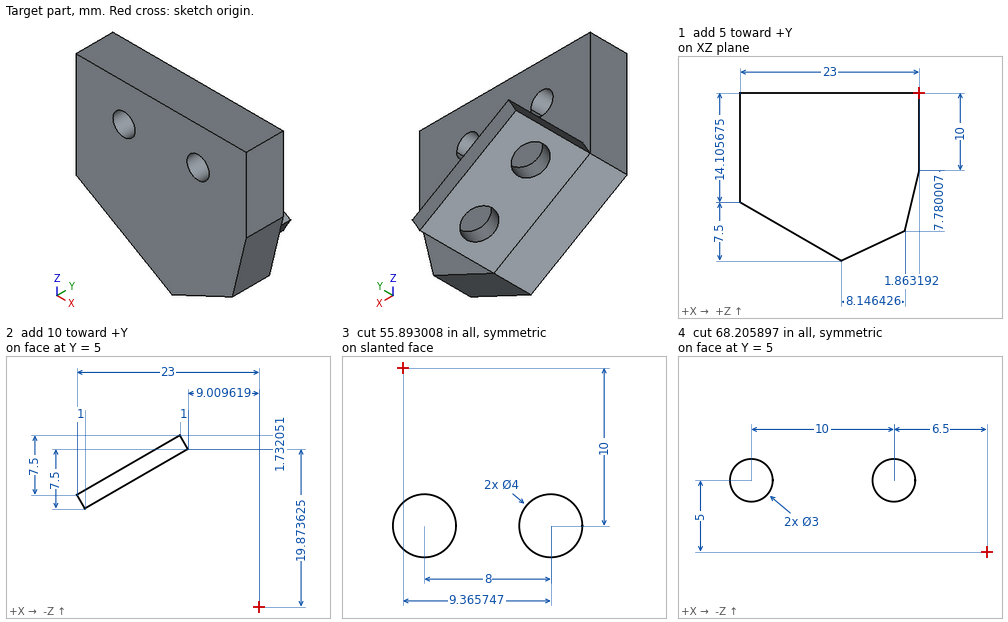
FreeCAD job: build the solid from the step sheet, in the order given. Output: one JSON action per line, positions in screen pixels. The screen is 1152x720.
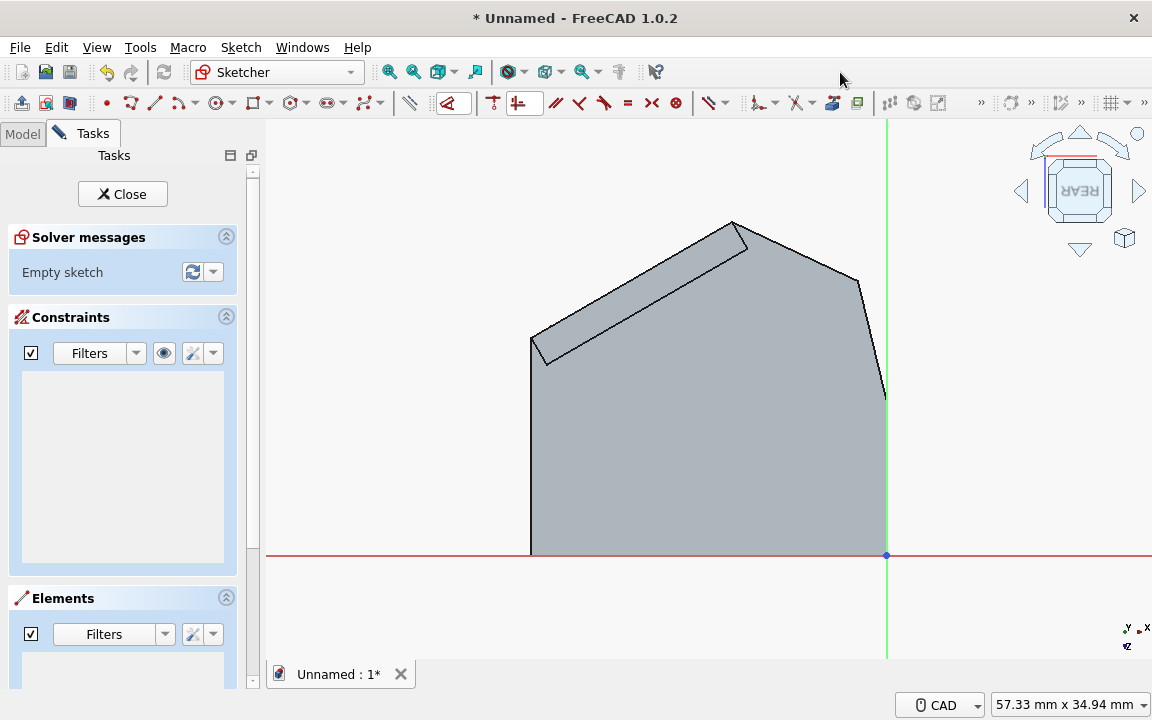
{"action": "scroll", "coordinate": [878, 631], "scroll_direction": "up", "scroll_amount": 3}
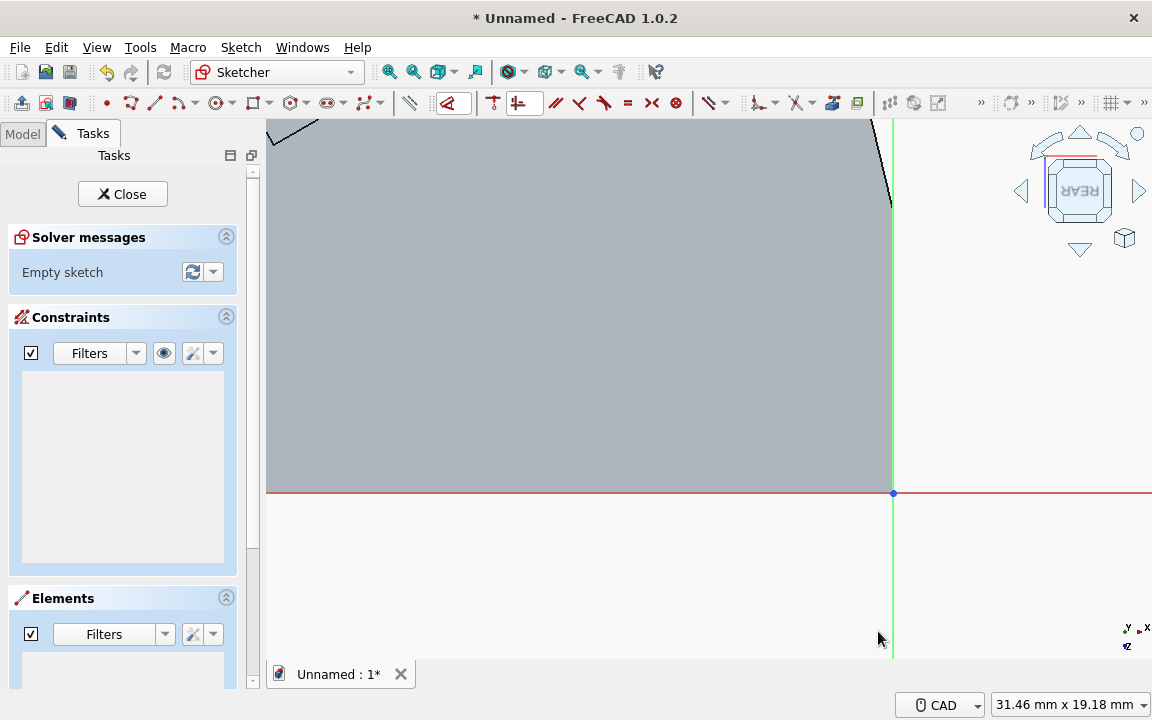
{"action": "left_click", "coordinate": [216, 104]}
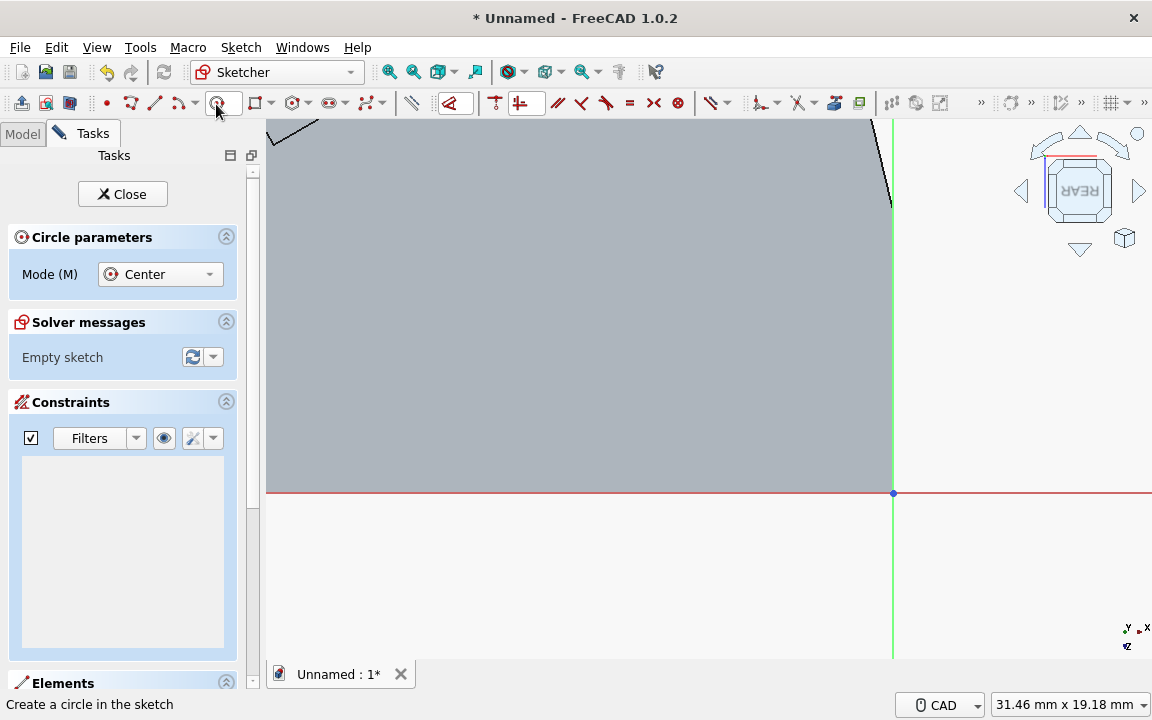
{"action": "left_click", "coordinate": [429, 353]}
{"action": "mouse_move", "coordinate": [459, 323]}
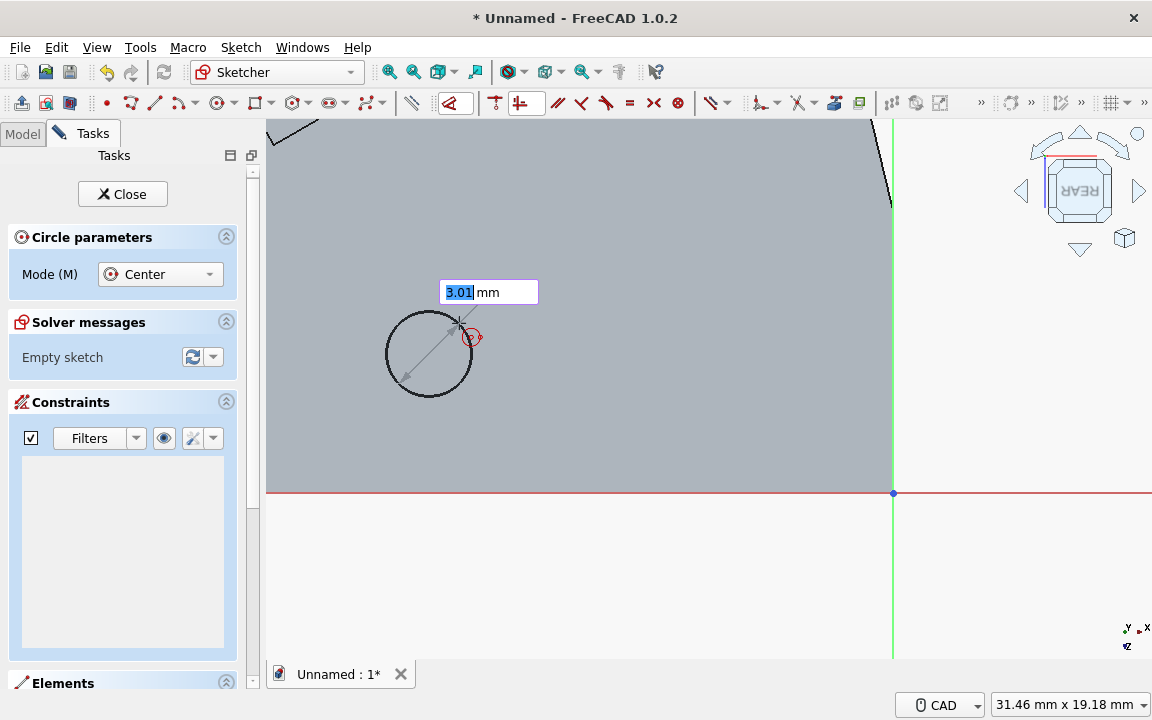
{"action": "type", "text": "3"}
{"action": "key", "text": "Return"}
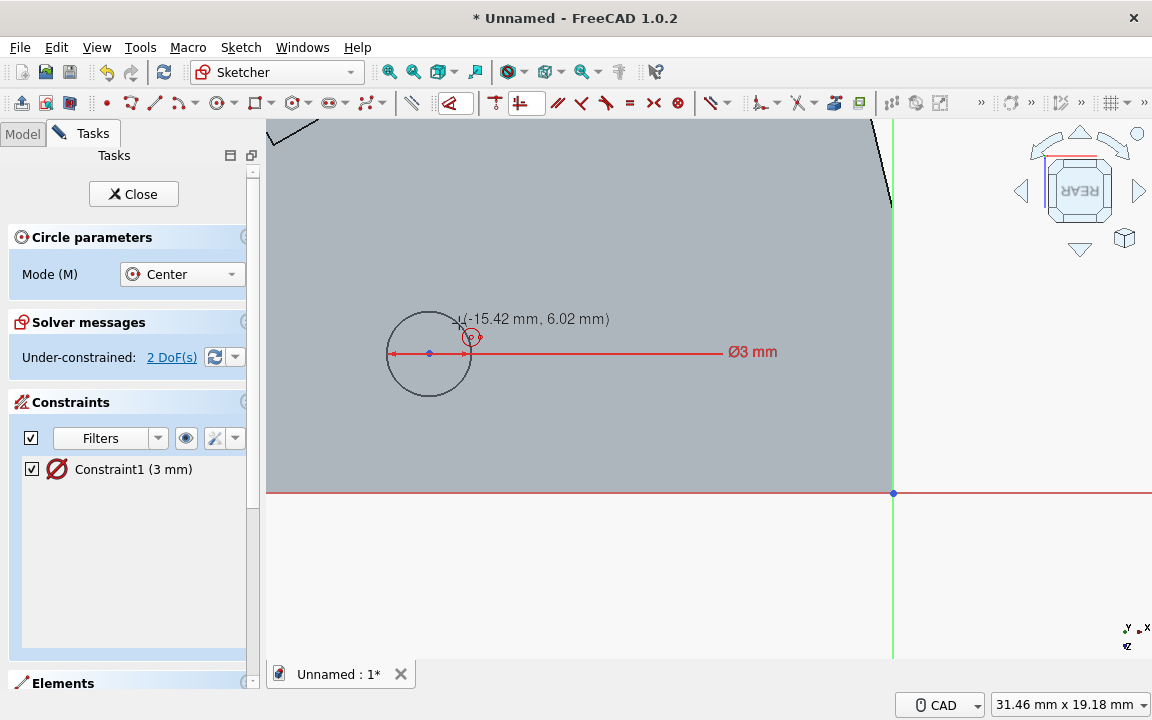
{"action": "left_click", "coordinate": [710, 353]}
{"action": "mouse_move", "coordinate": [740, 323]}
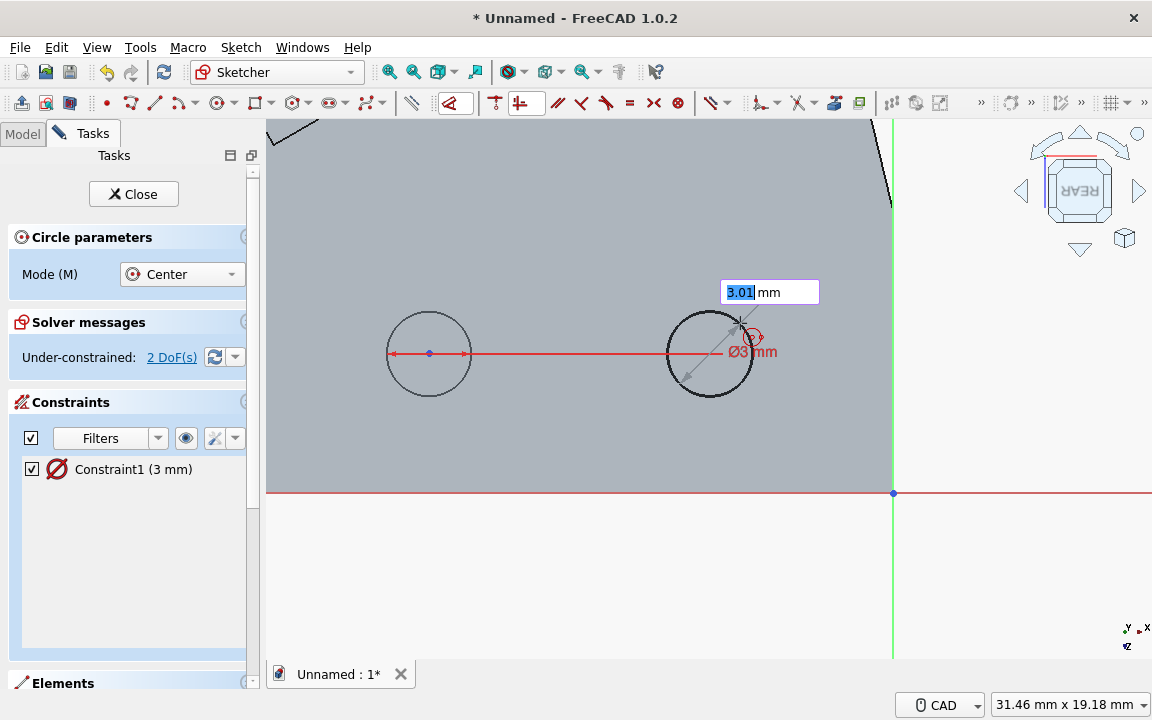
{"action": "type", "text": "3"}
{"action": "key", "text": "Return"}
{"action": "key", "text": "Escape"}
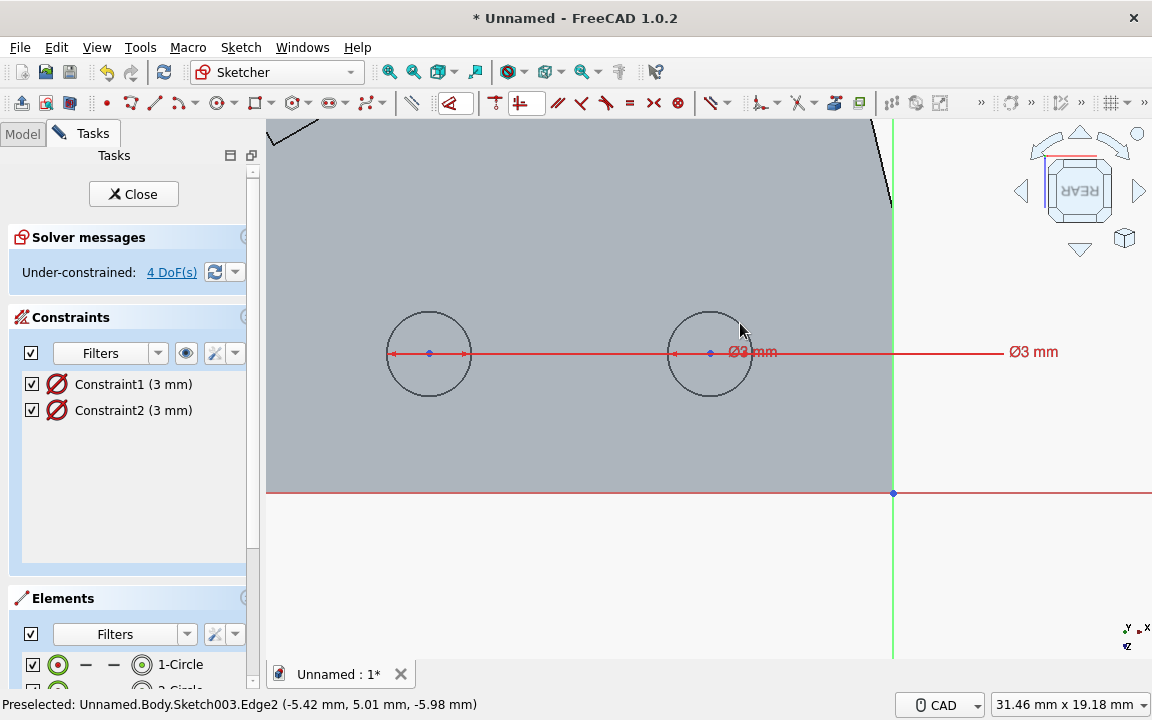
{"action": "left_click", "coordinate": [429, 354]}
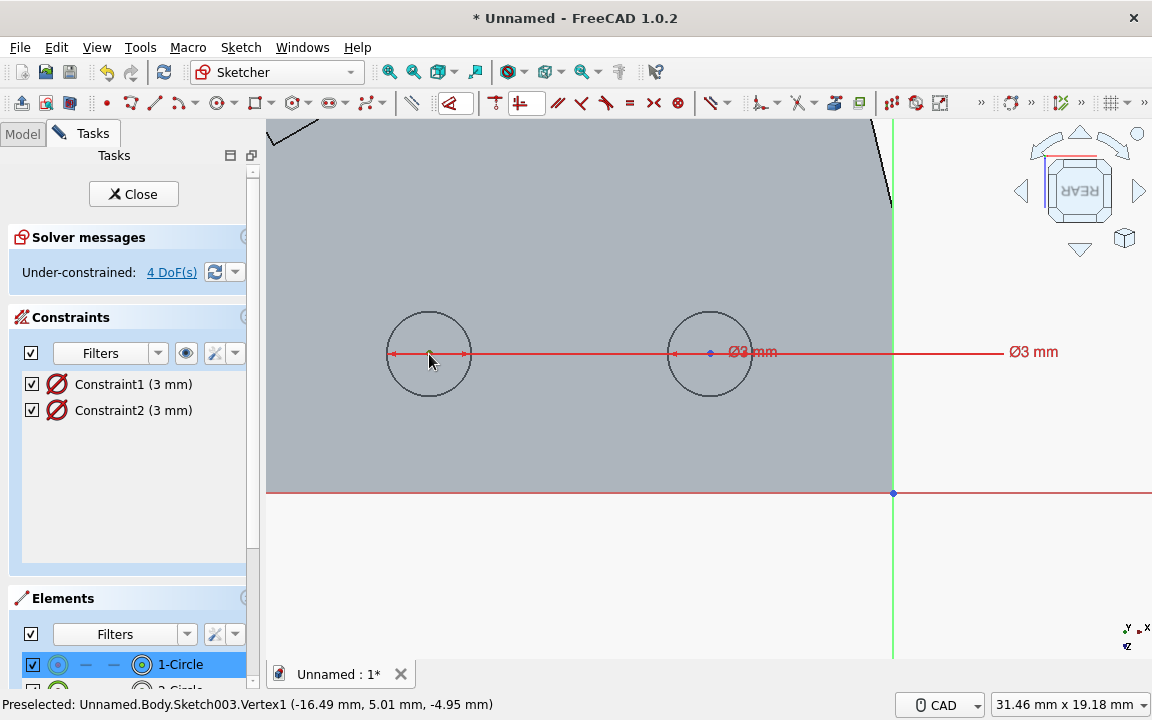
{"action": "left_click", "coordinate": [710, 354]}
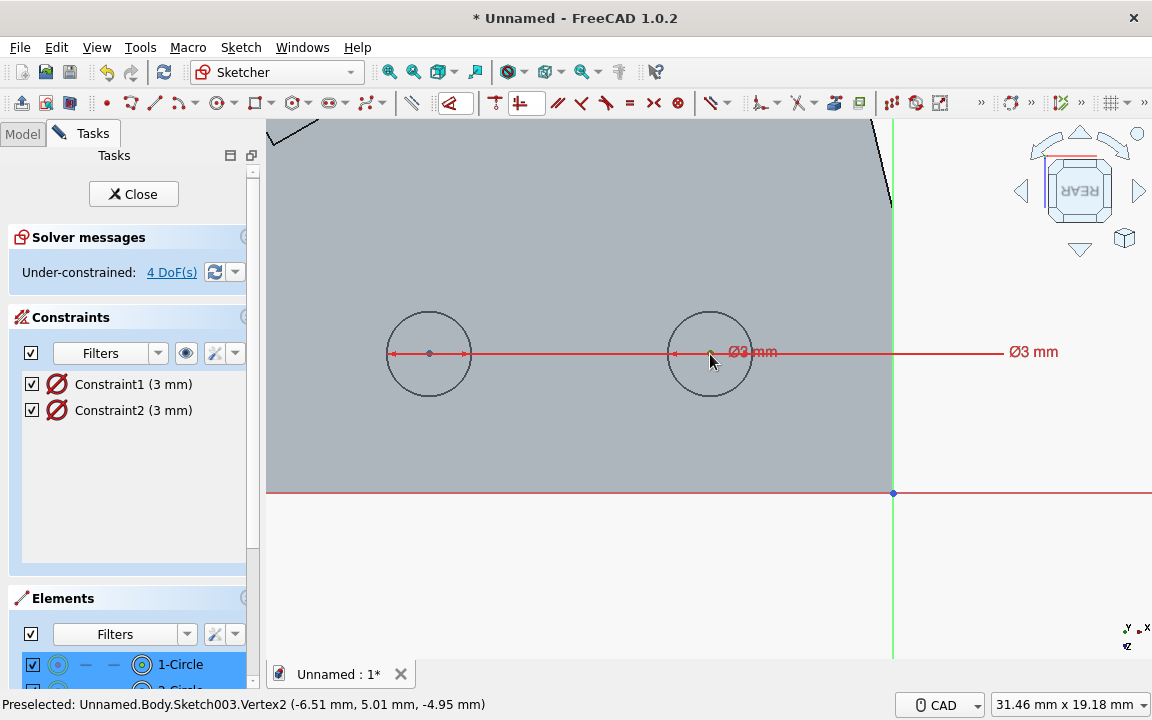
{"action": "left_click", "coordinate": [540, 104]}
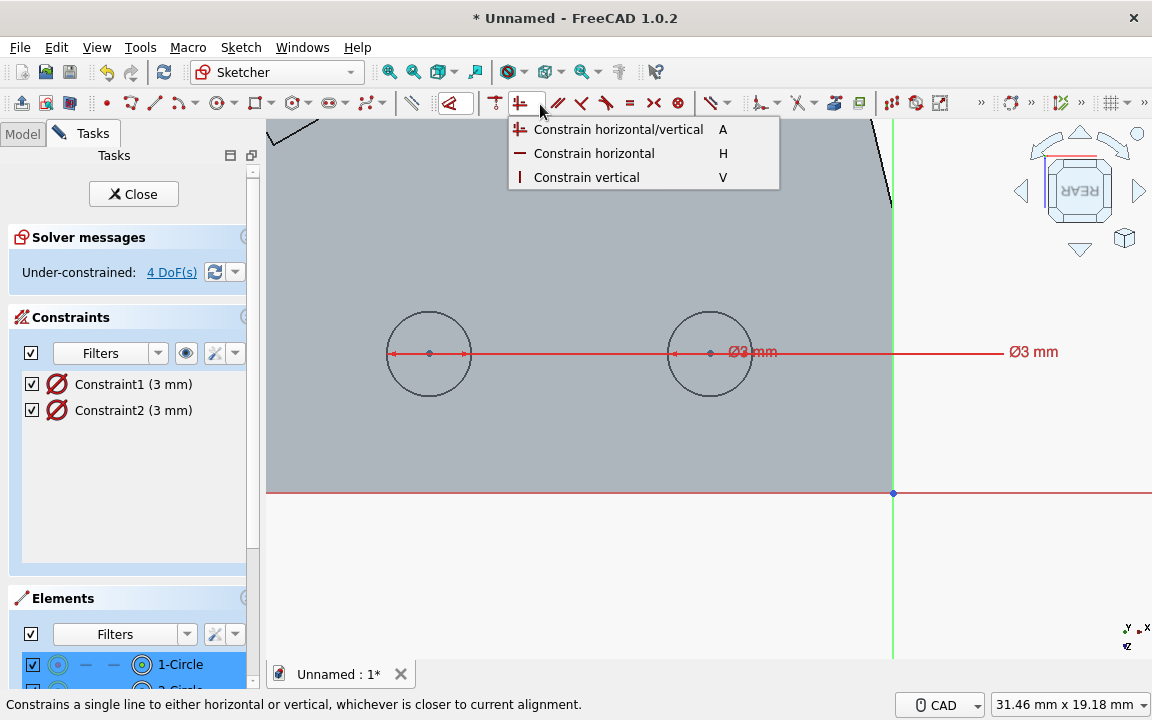
{"action": "left_click", "coordinate": [644, 153]}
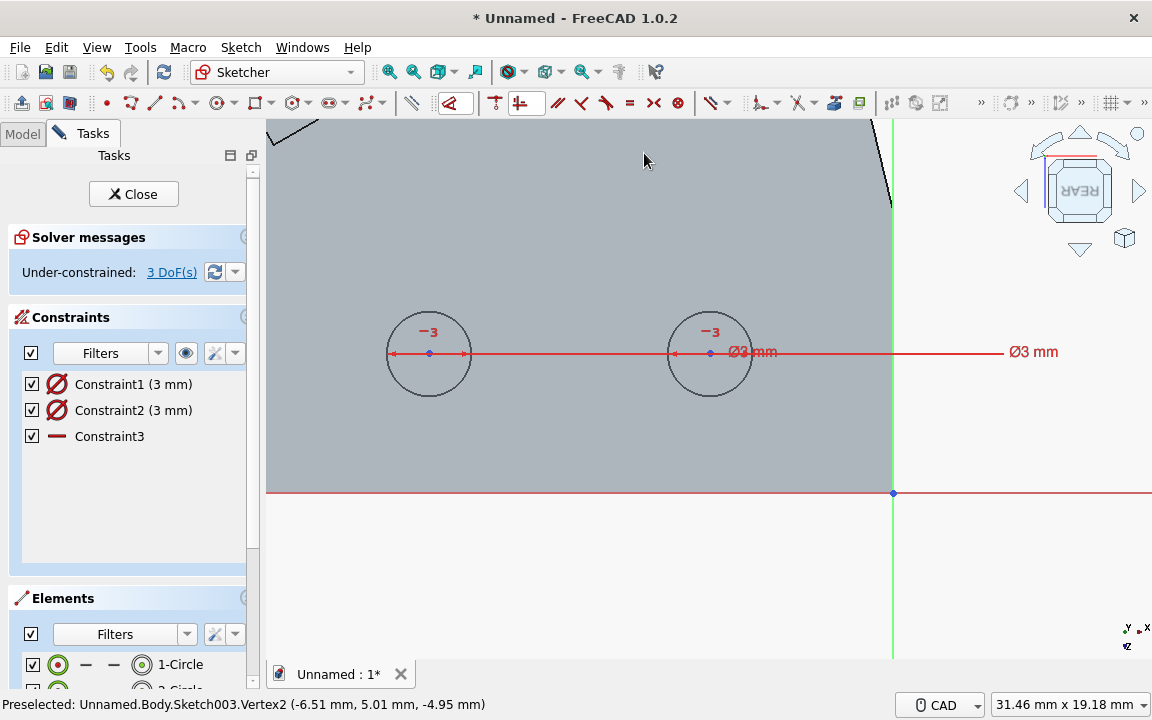
{"action": "left_click", "coordinate": [429, 354]}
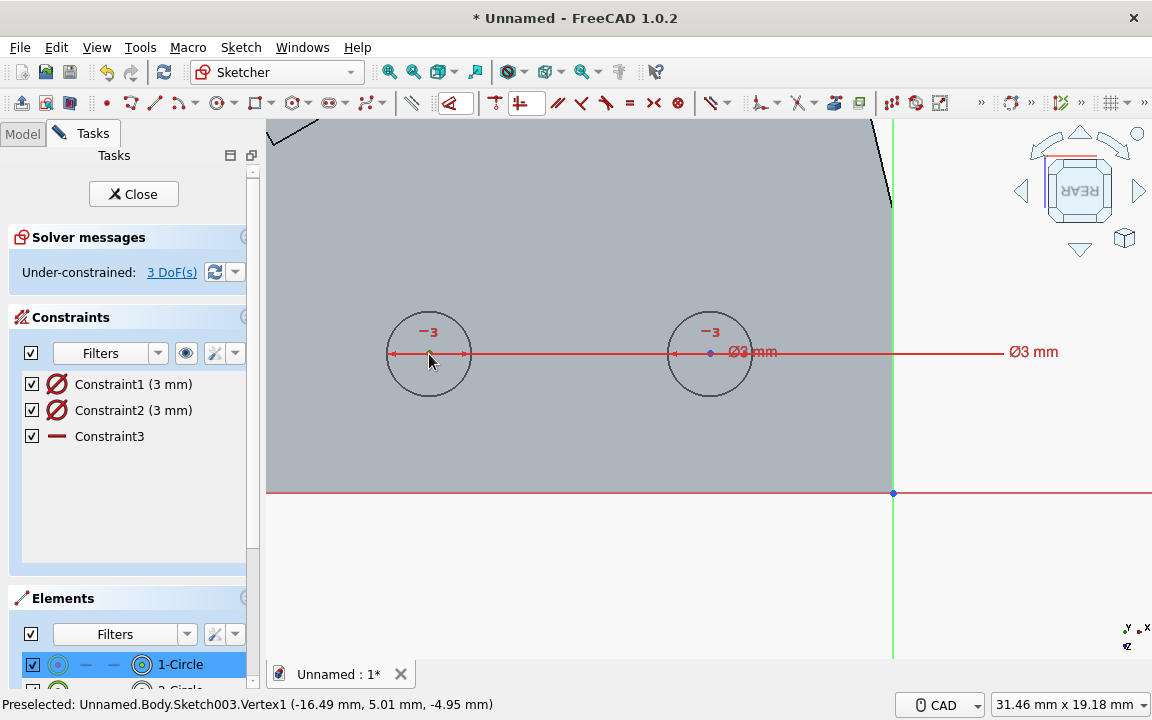
{"action": "key", "text": "i"}